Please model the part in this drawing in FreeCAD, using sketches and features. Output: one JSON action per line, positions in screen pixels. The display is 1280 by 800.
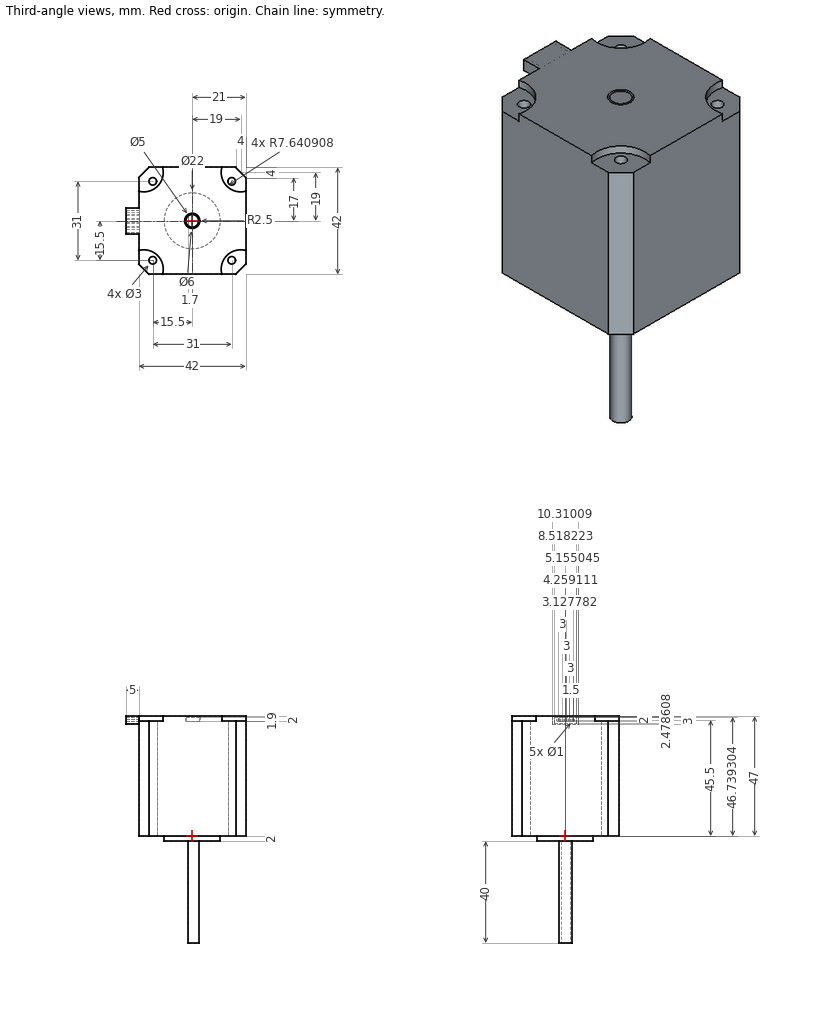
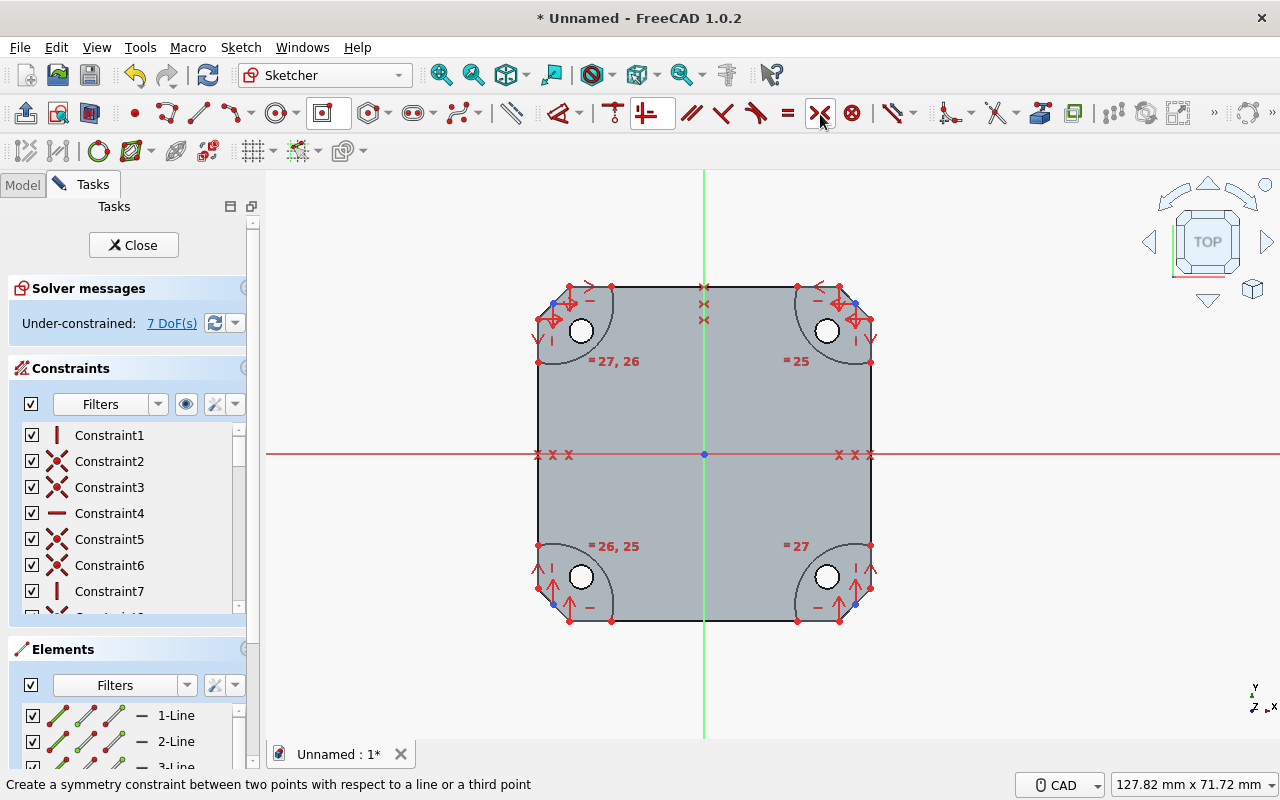
{"action": "left_click", "coordinate": [558, 114]}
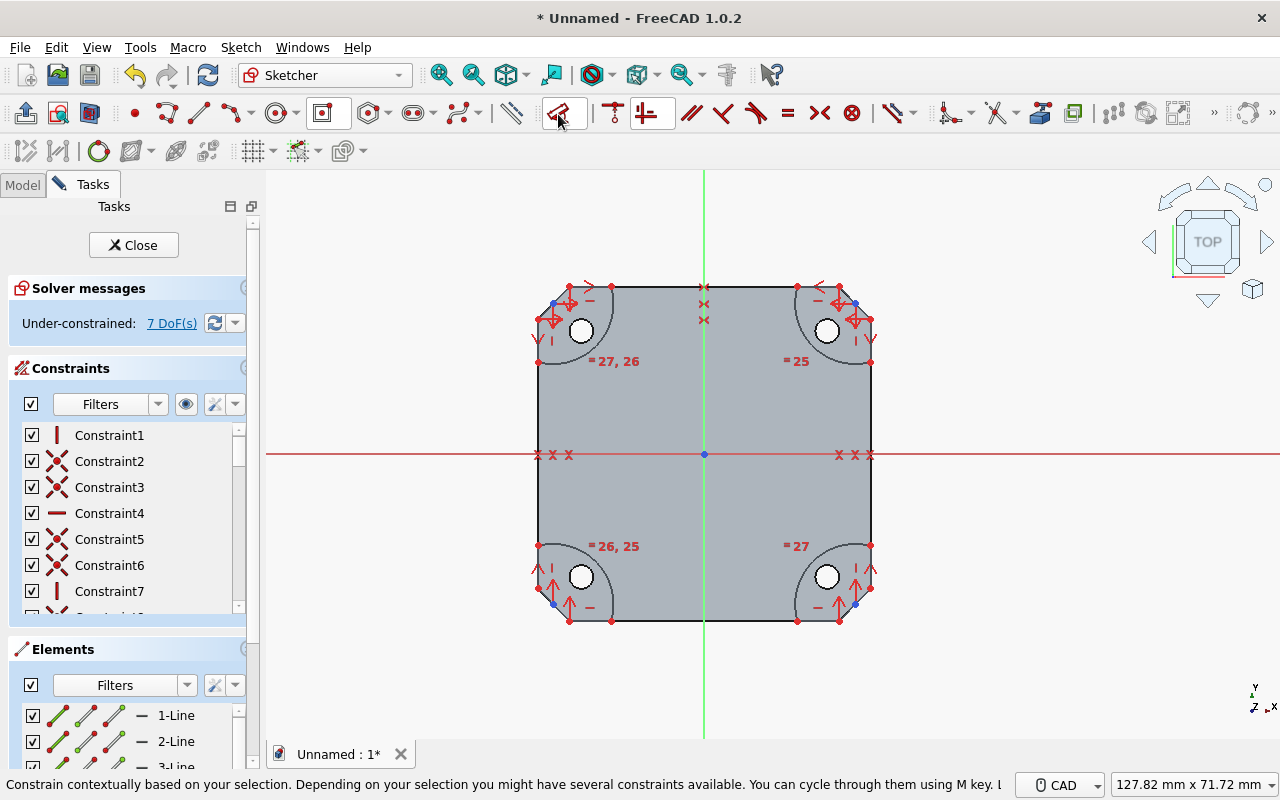
{"action": "left_click", "coordinate": [799, 324]}
{"action": "left_click", "coordinate": [769, 335]}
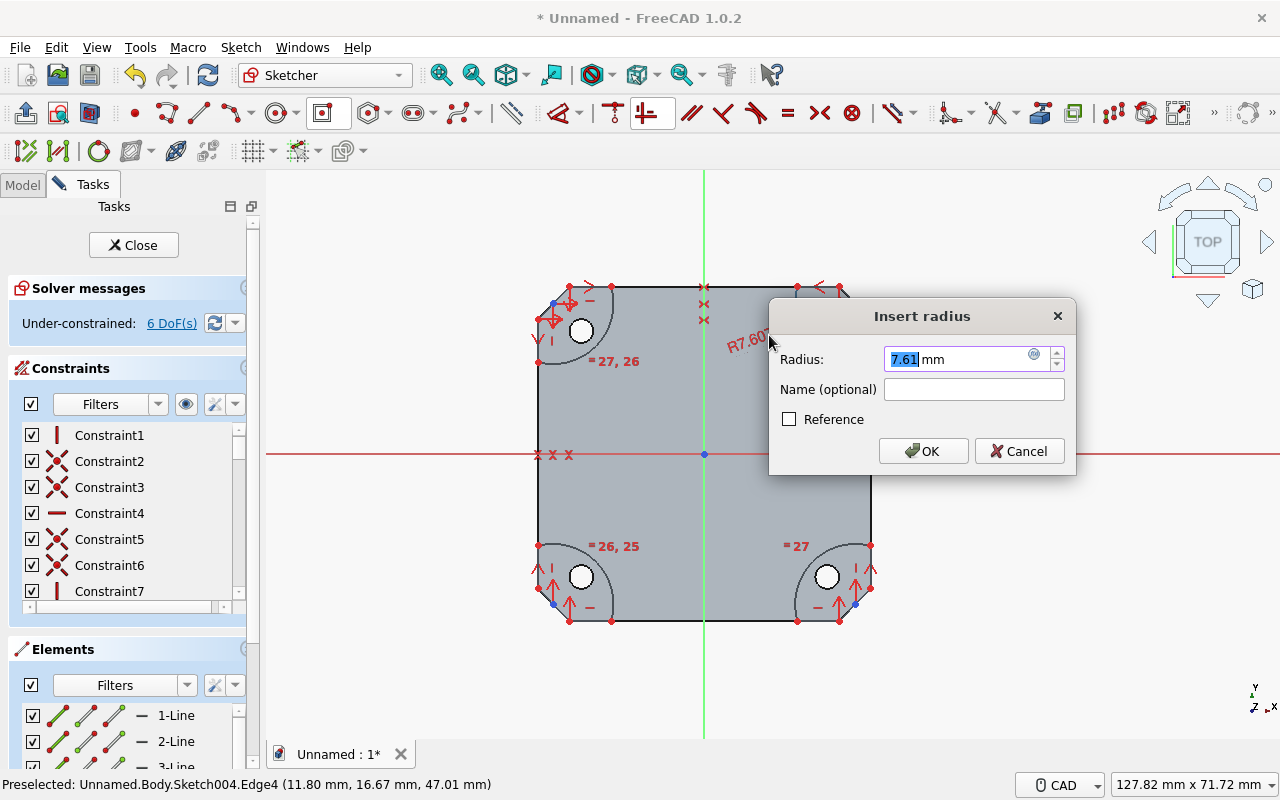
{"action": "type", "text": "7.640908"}
{"action": "key", "text": "Return"}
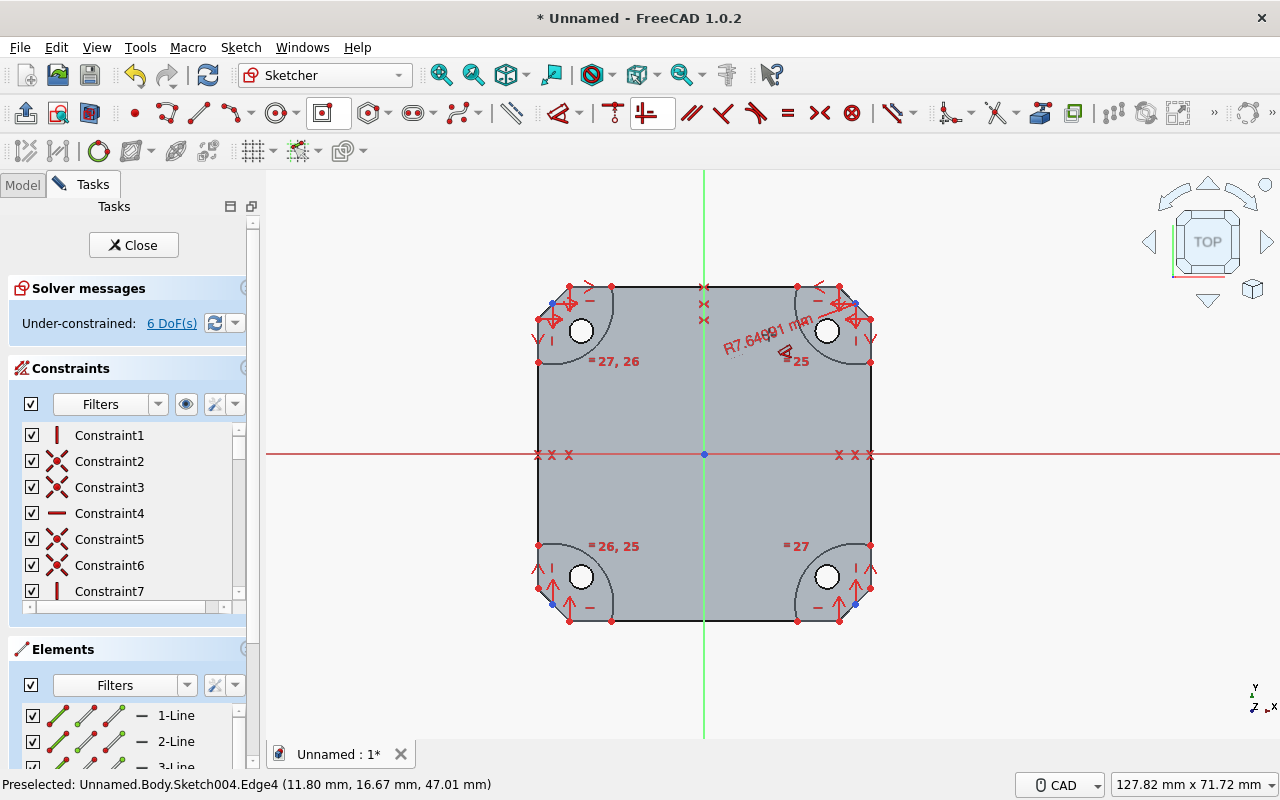
{"action": "scroll", "coordinate": [861, 310], "scroll_direction": "up", "scroll_amount": 2}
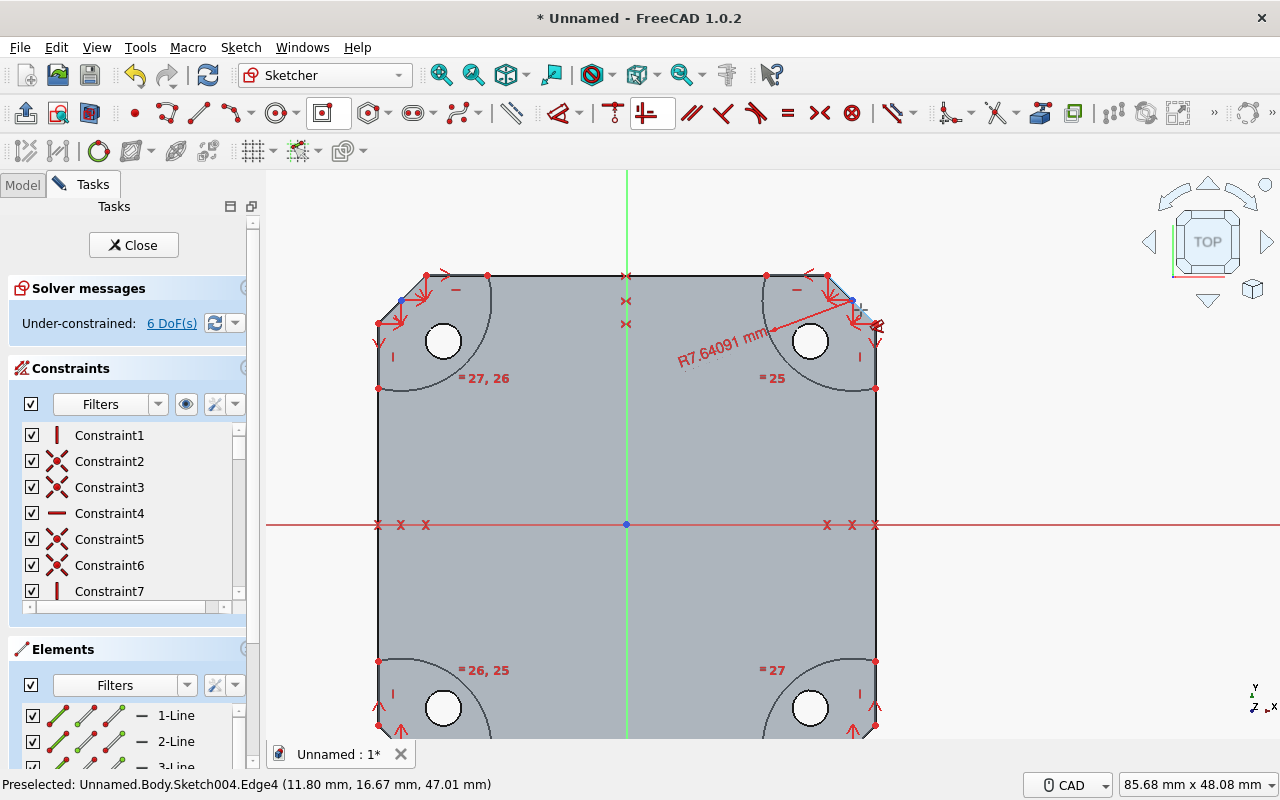
{"action": "left_click", "coordinate": [861, 309]}
{"action": "left_click", "coordinate": [851, 241]}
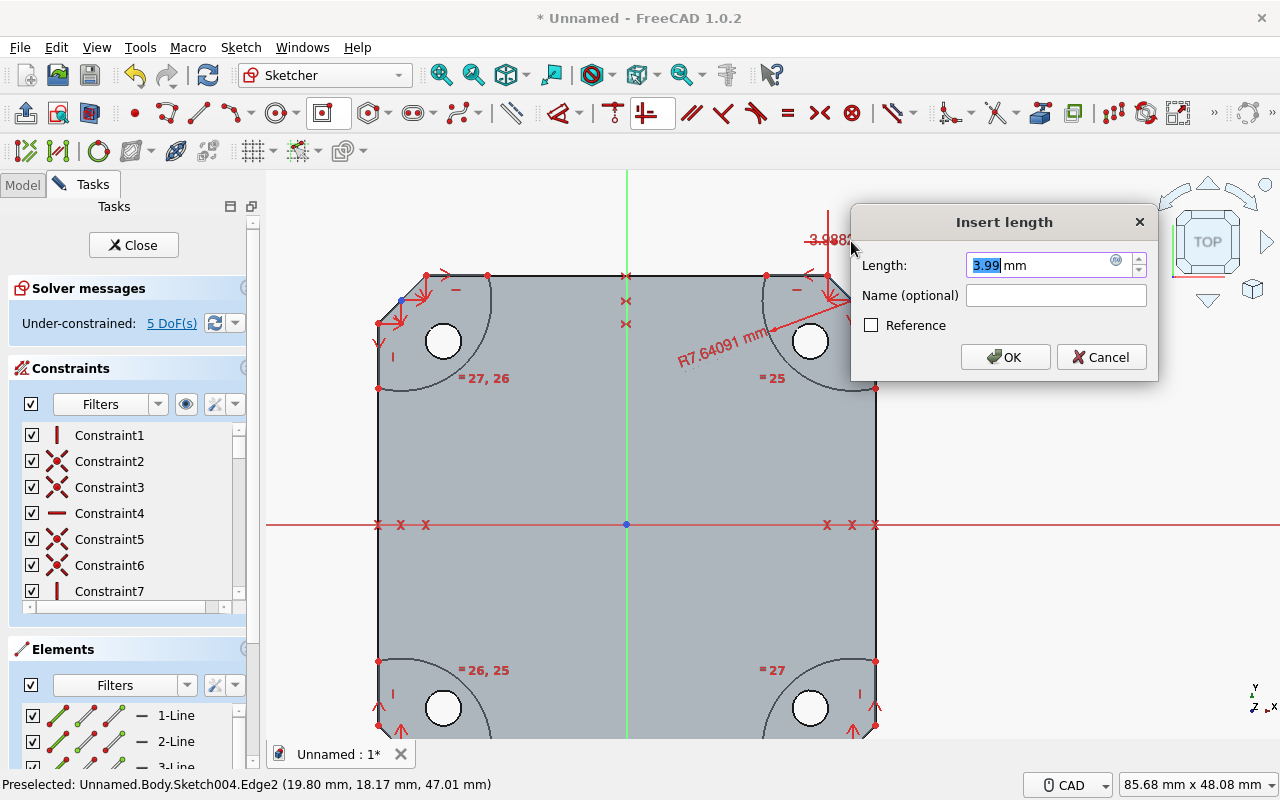
{"action": "type", "text": "4"}
{"action": "key", "text": "Return"}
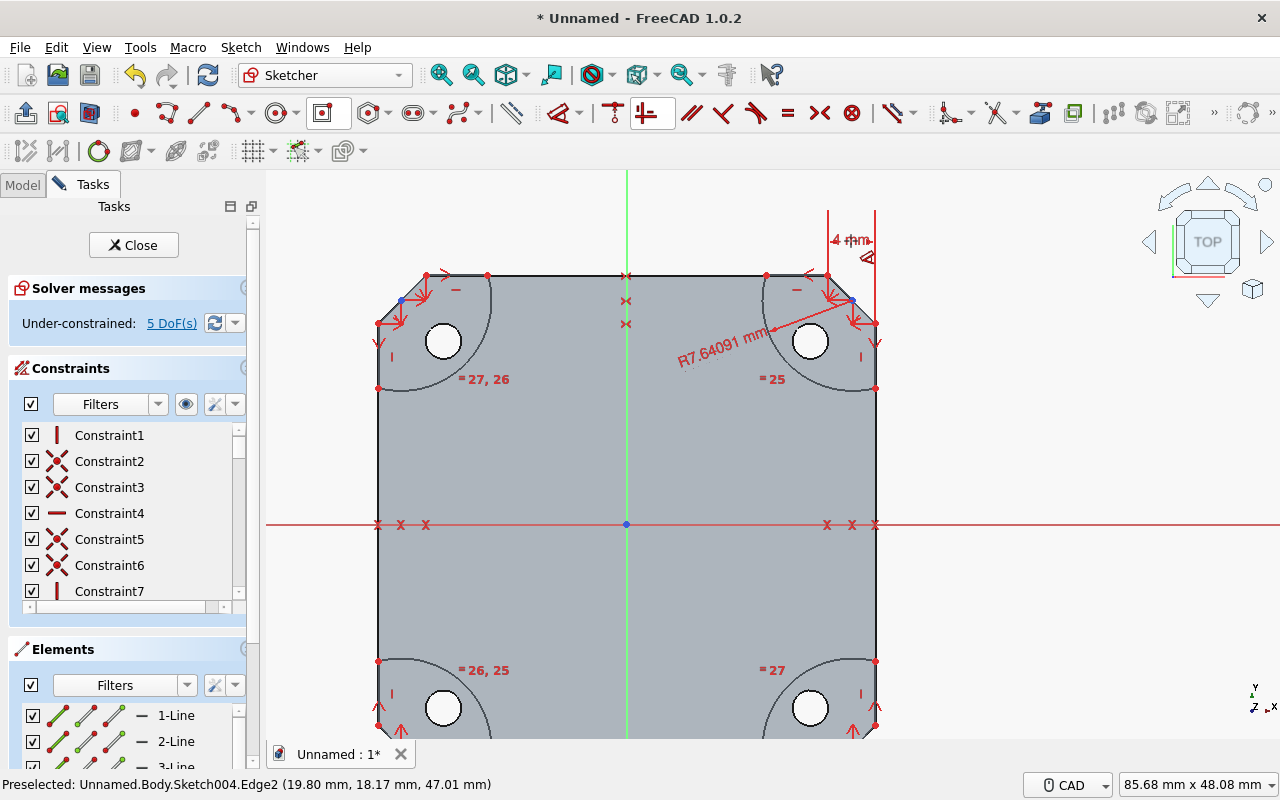
{"action": "left_click", "coordinate": [861, 309]}
{"action": "left_click", "coordinate": [909, 300]}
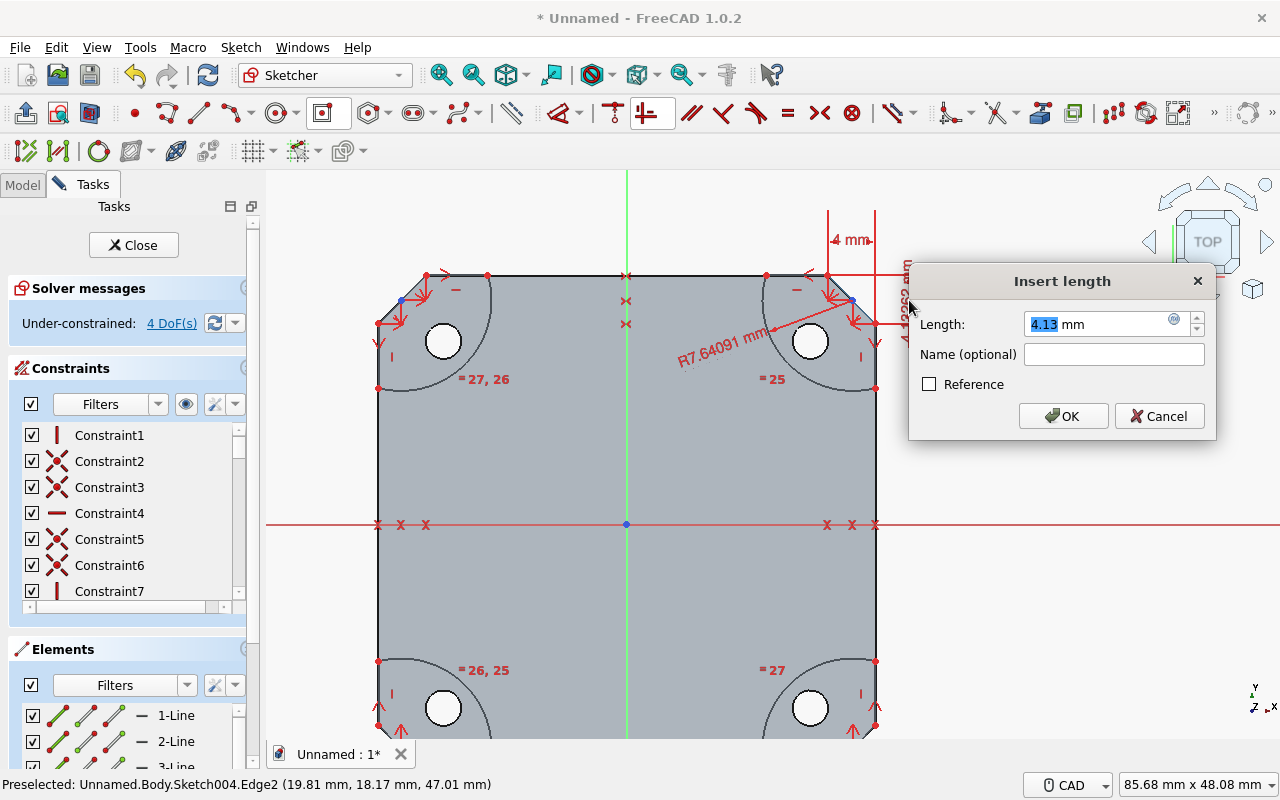
{"action": "type", "text": "4"}
{"action": "key", "text": "Return"}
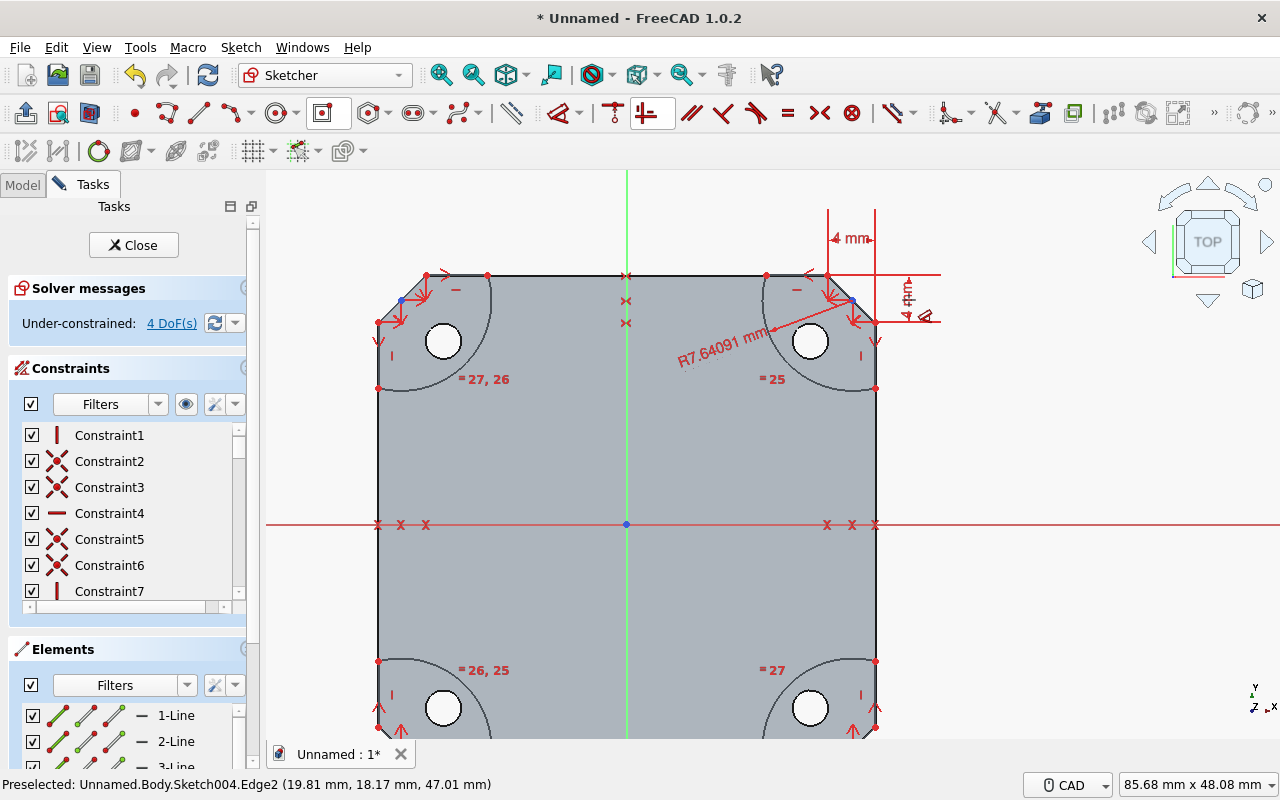
{"action": "left_click", "coordinate": [875, 388]}
{"action": "left_click", "coordinate": [808, 354]}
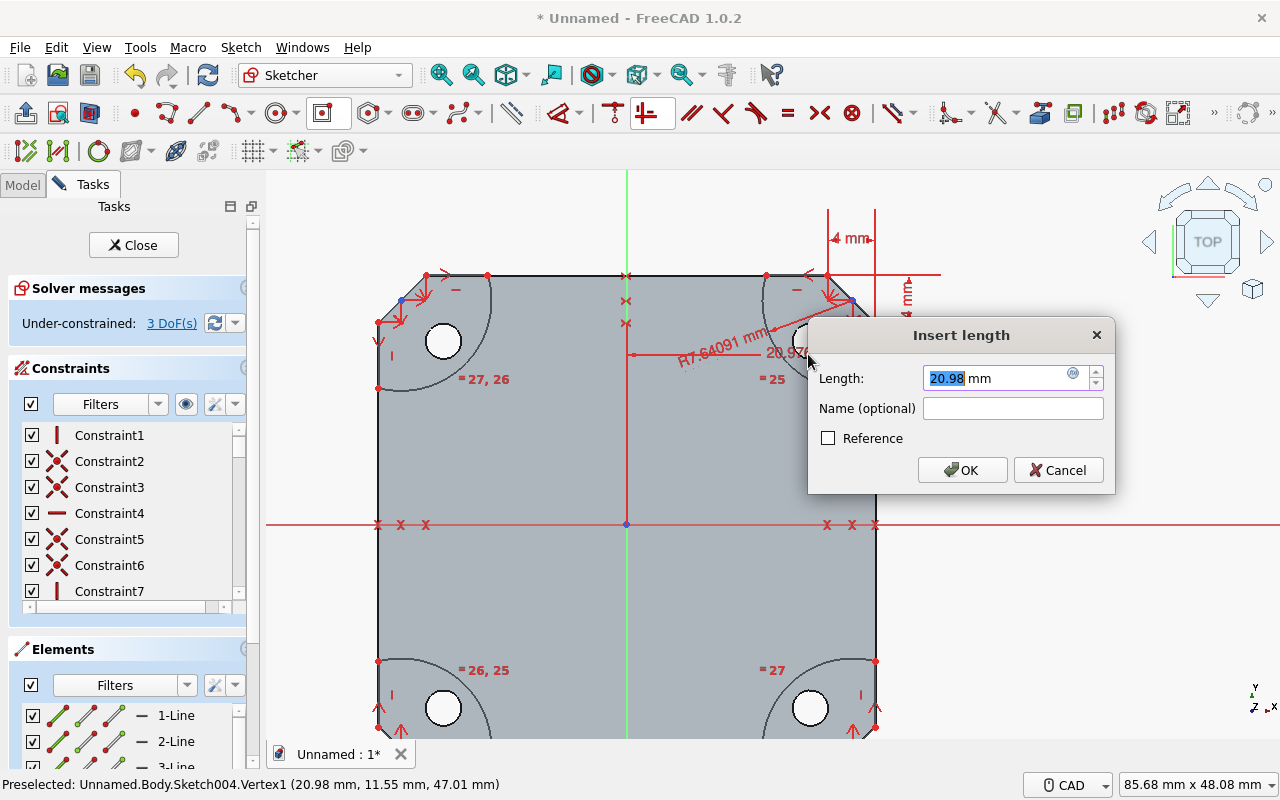
{"action": "type", "text": "21"}
{"action": "key", "text": "Return"}